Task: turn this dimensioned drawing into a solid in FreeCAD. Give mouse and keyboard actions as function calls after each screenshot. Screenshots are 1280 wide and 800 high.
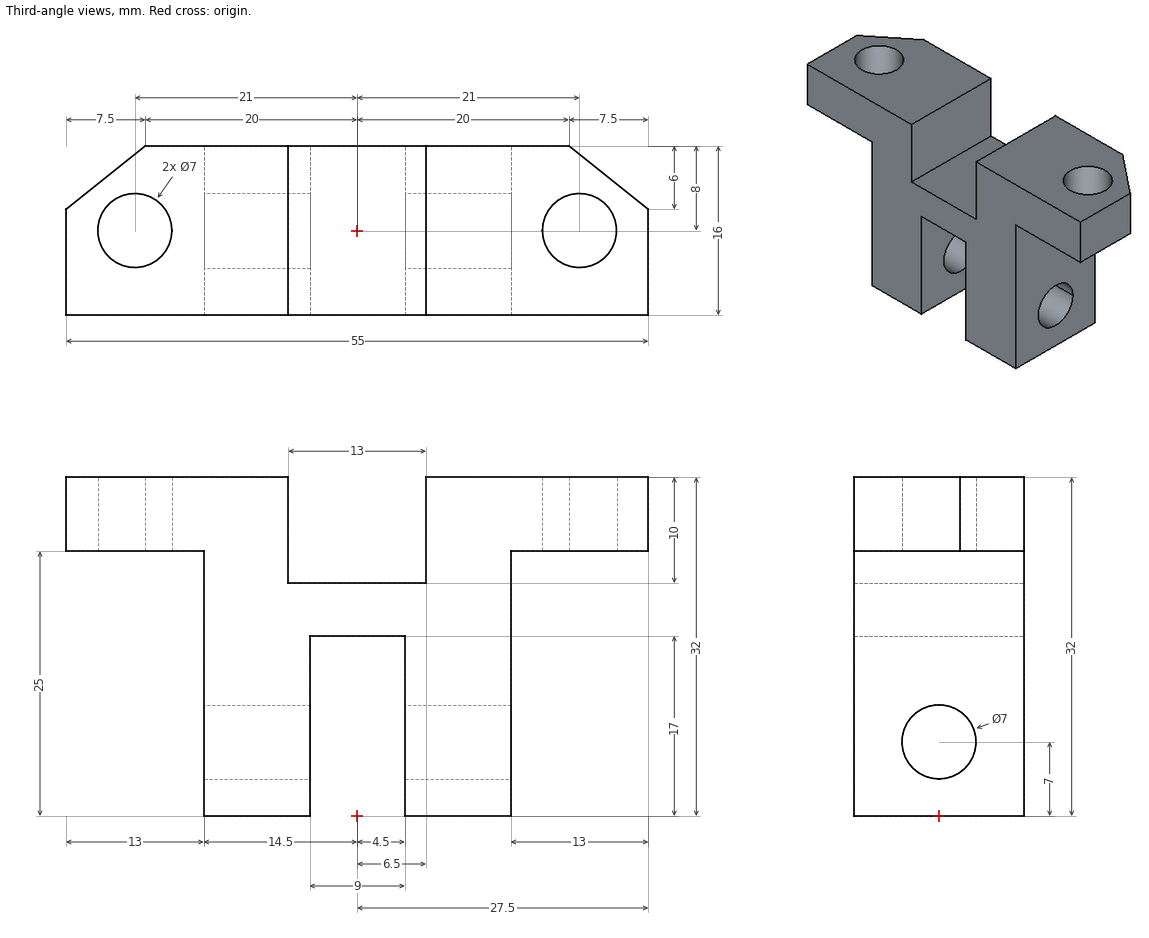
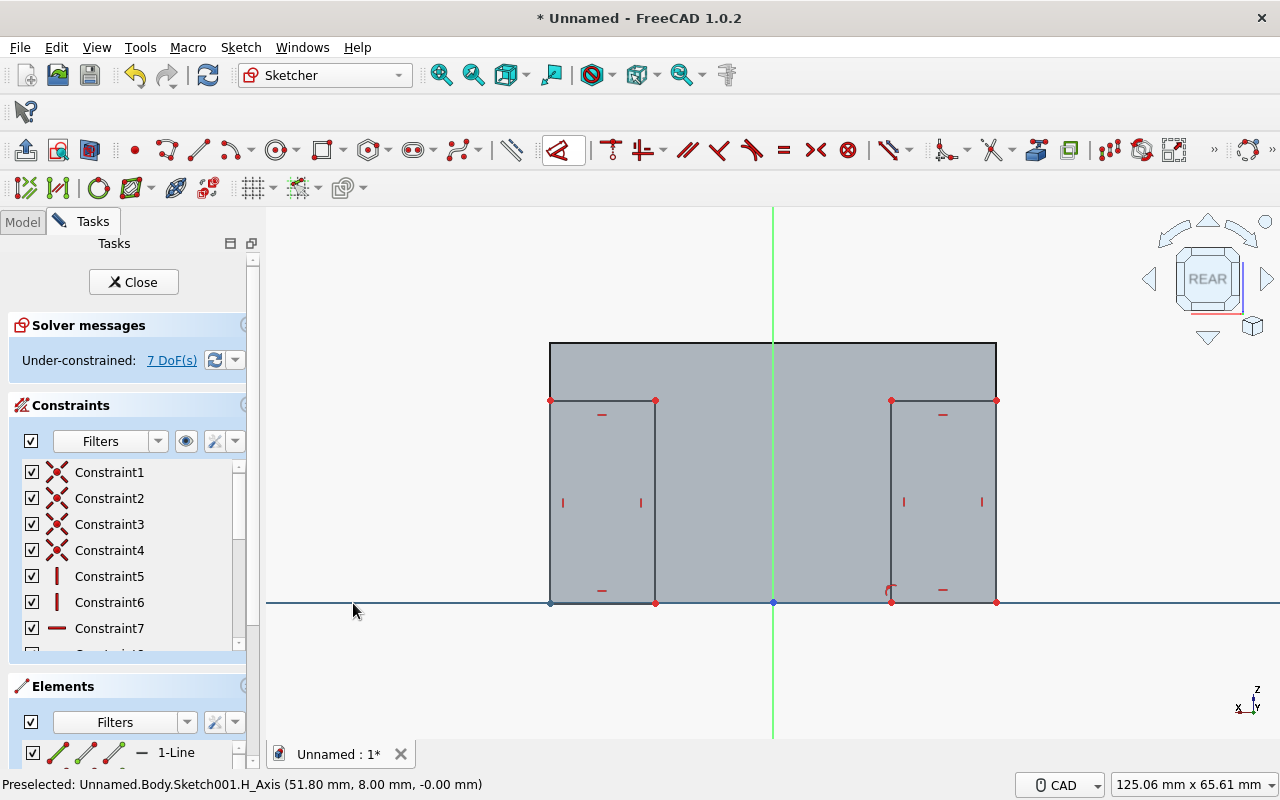
click(612, 150)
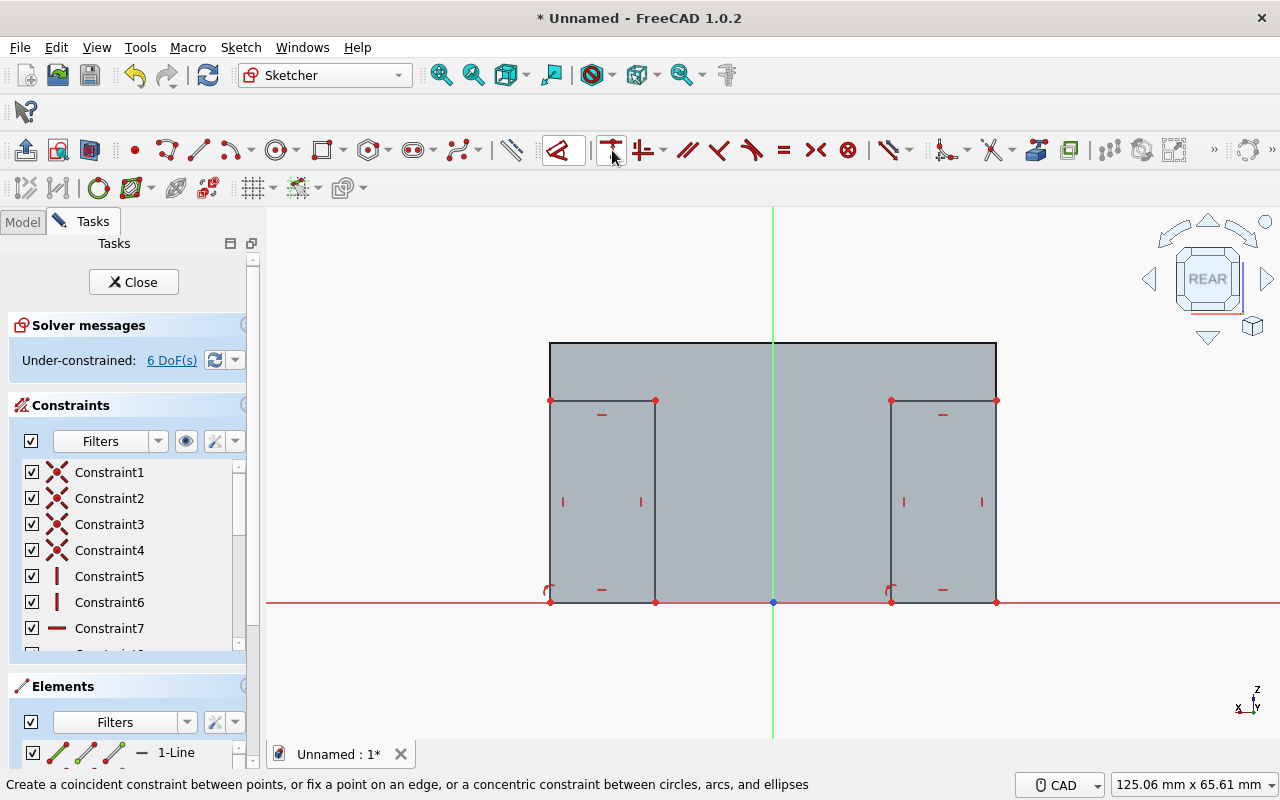
click(891, 462)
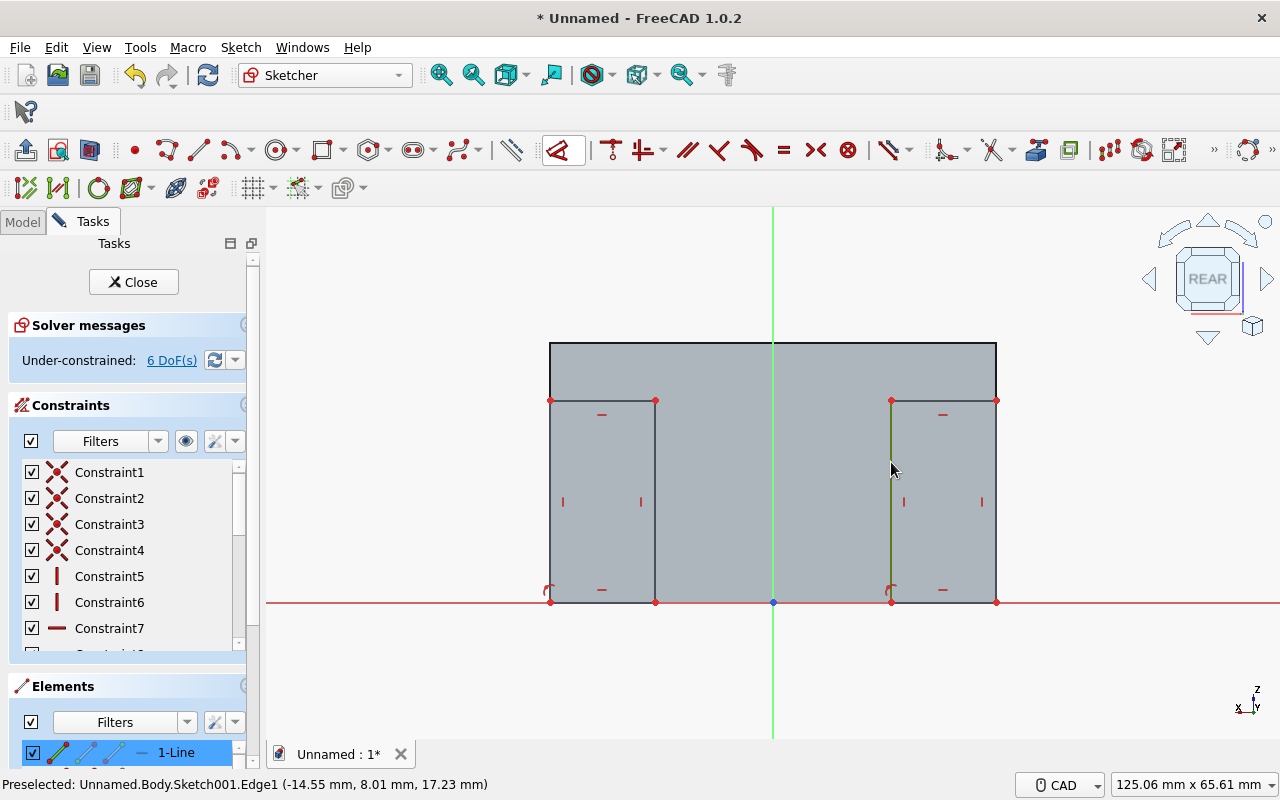
key(i)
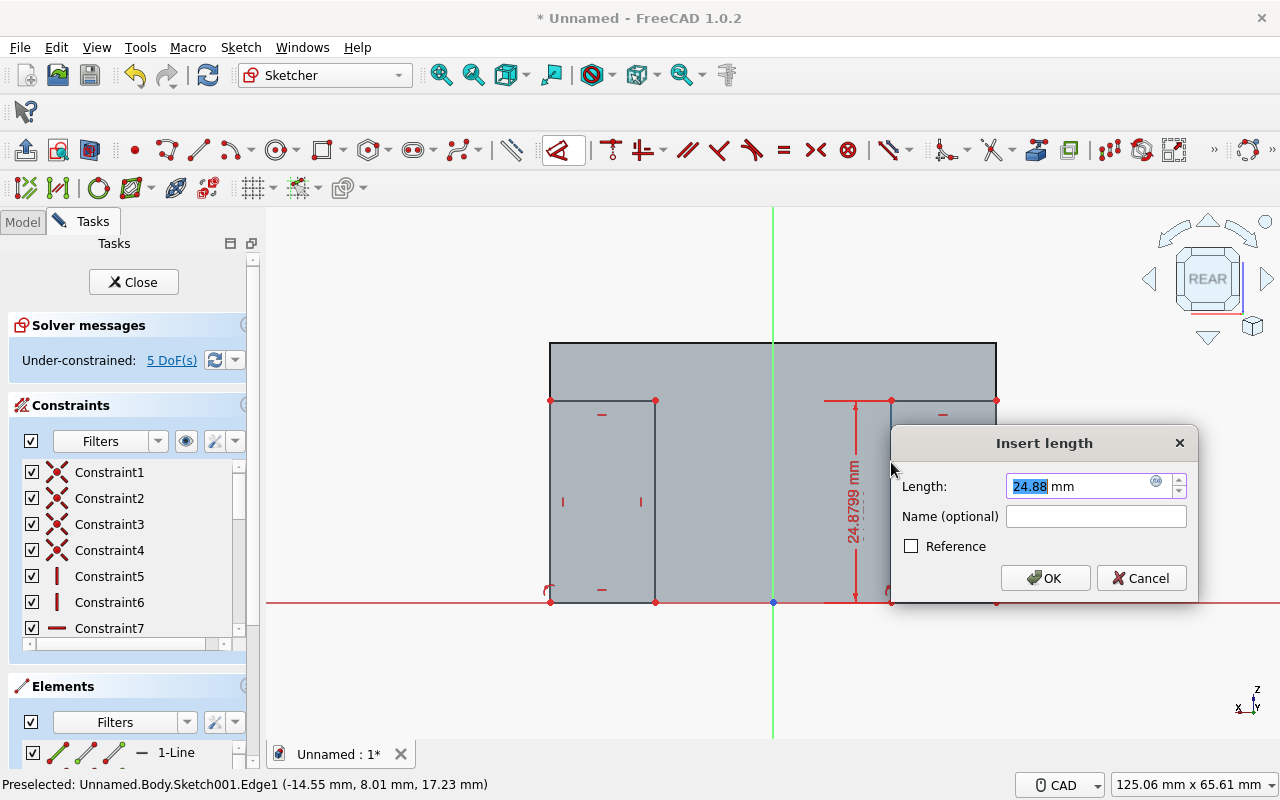
text(25)
key(Return)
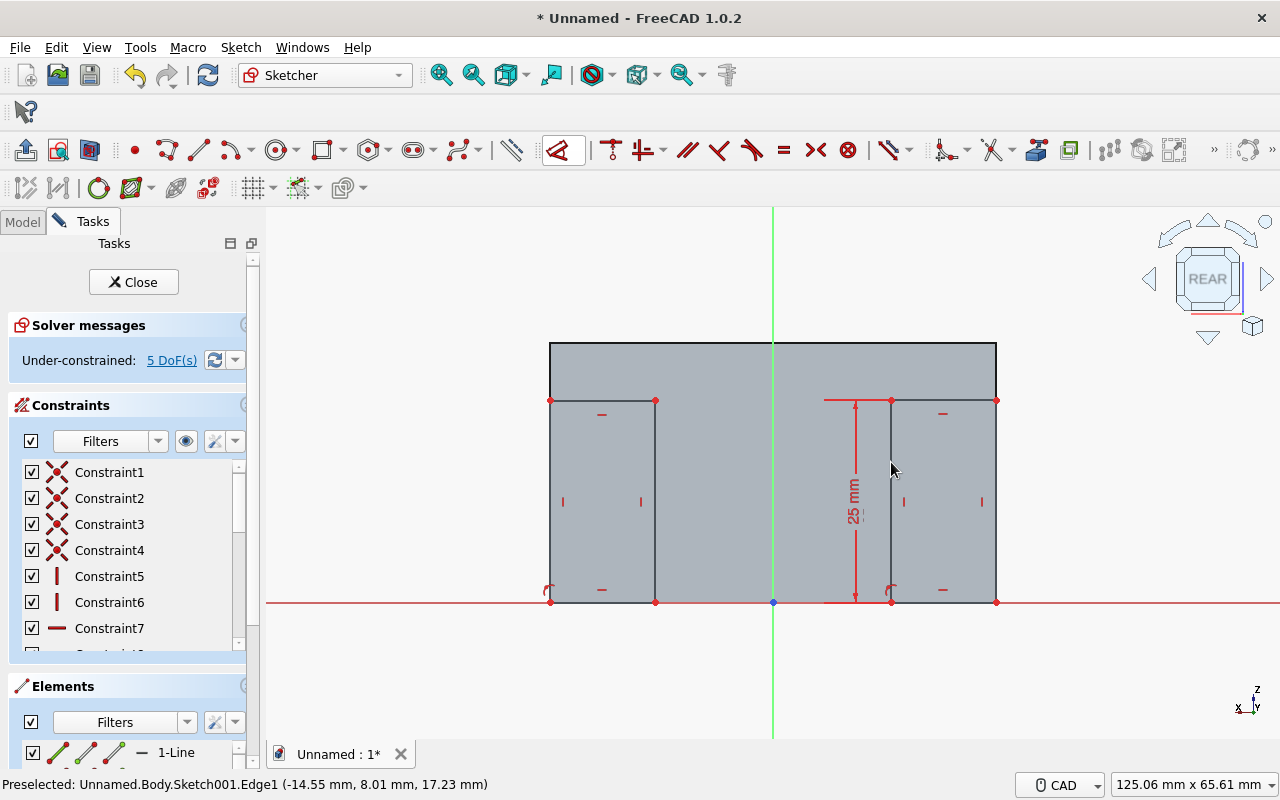
click(922, 603)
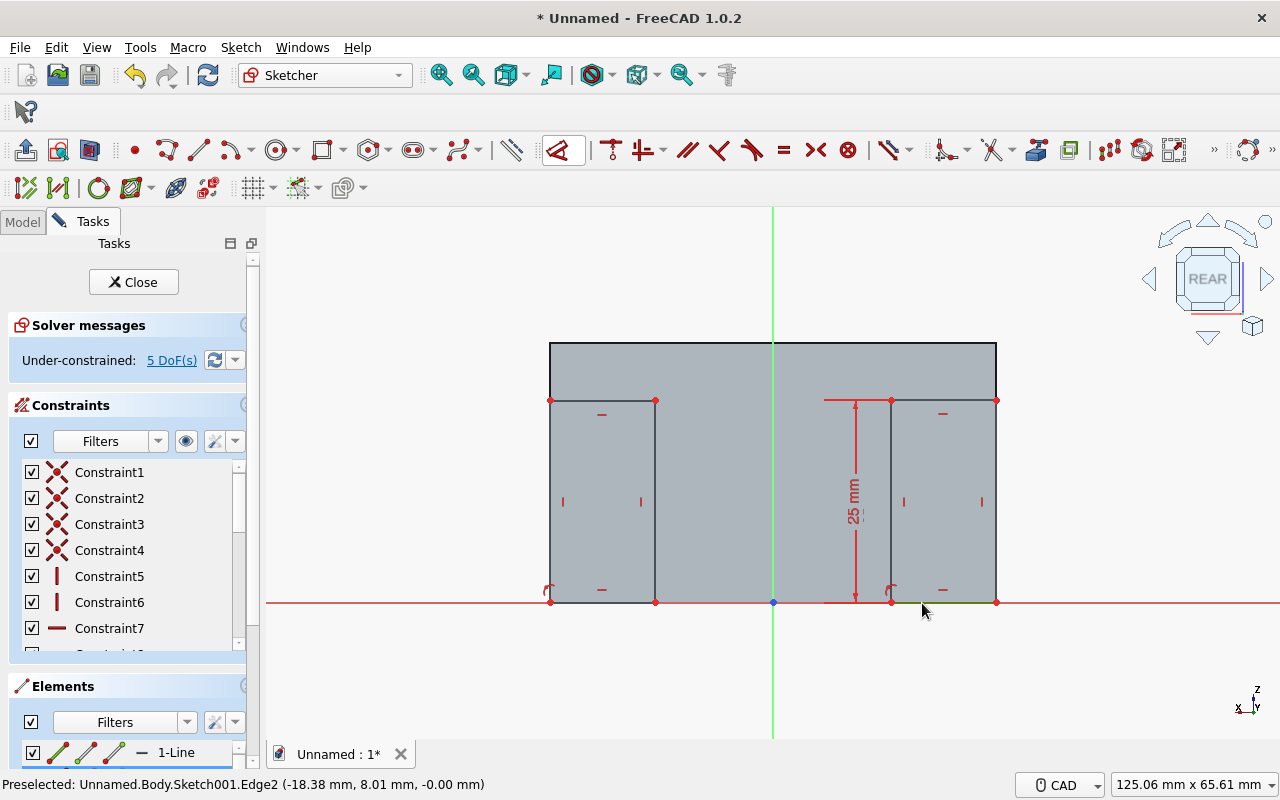
click(580, 150)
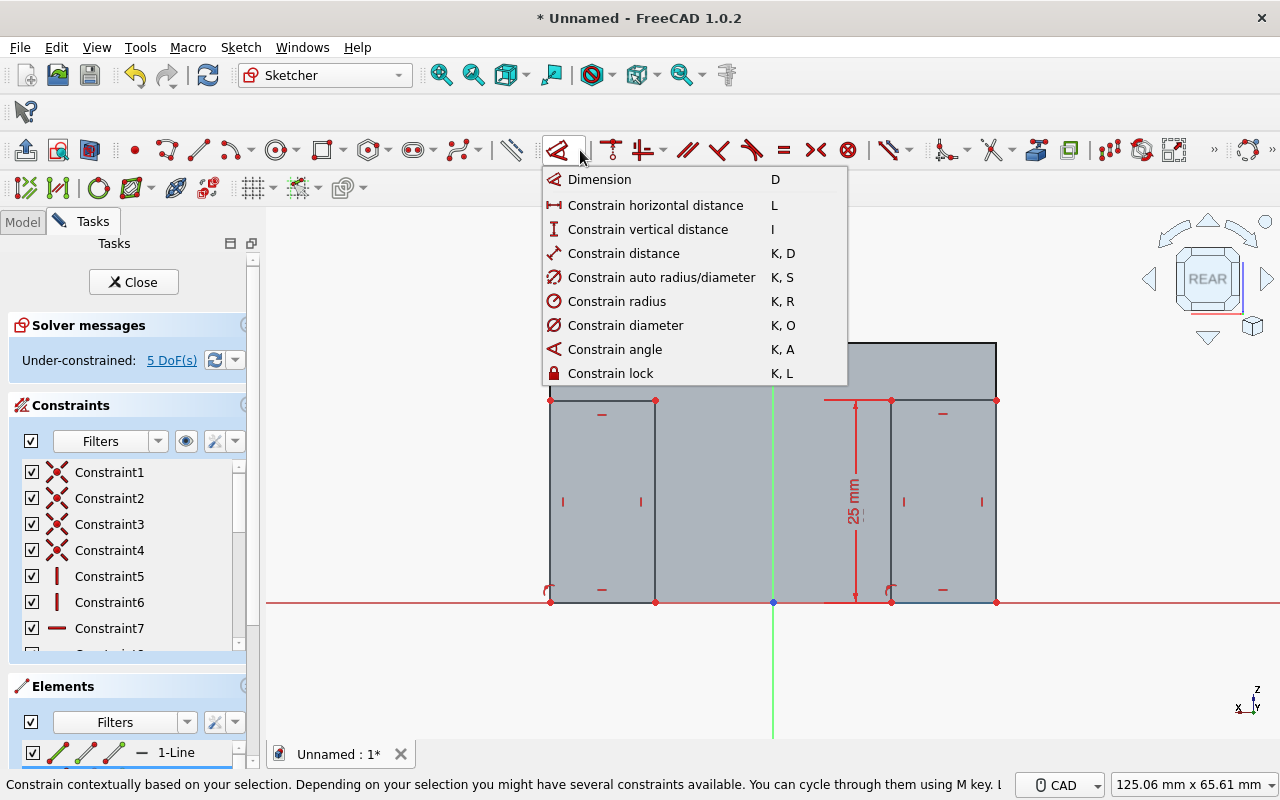
click(695, 205)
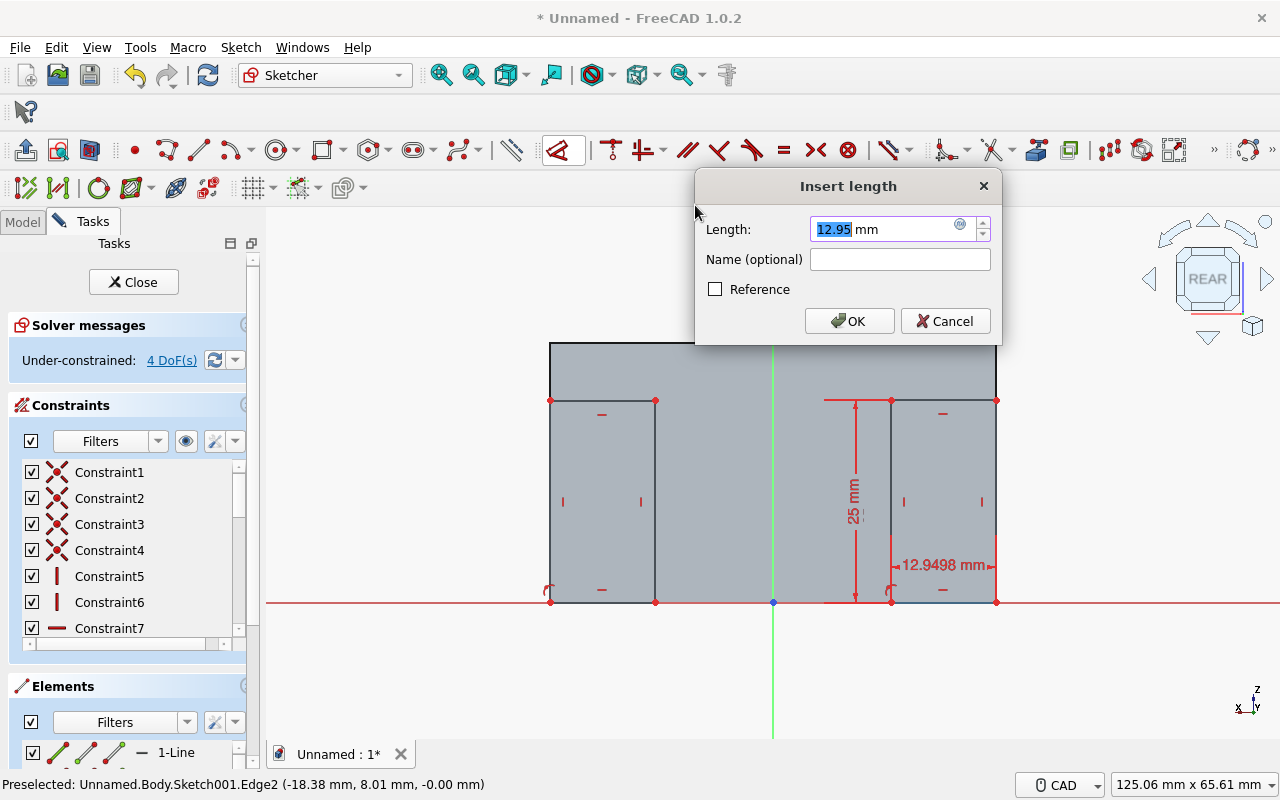
text(13)
key(Return)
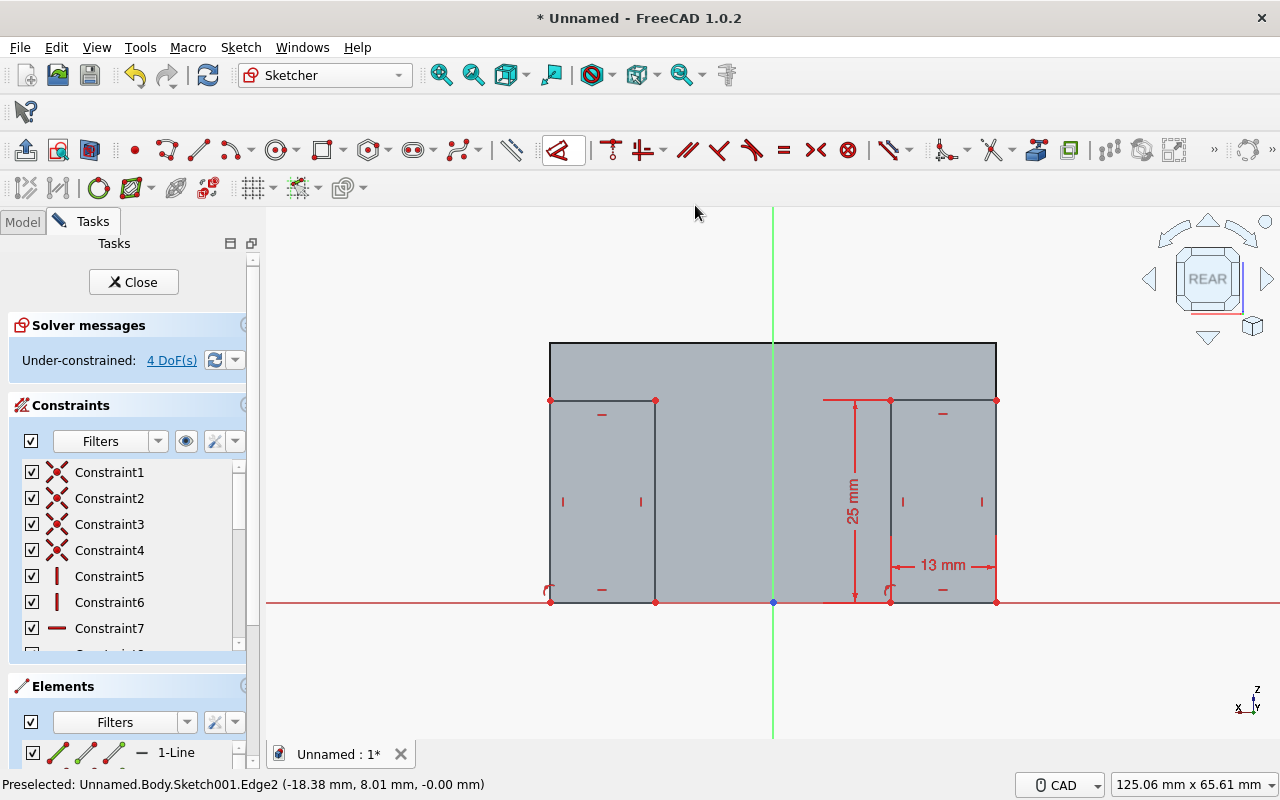
click(550, 462)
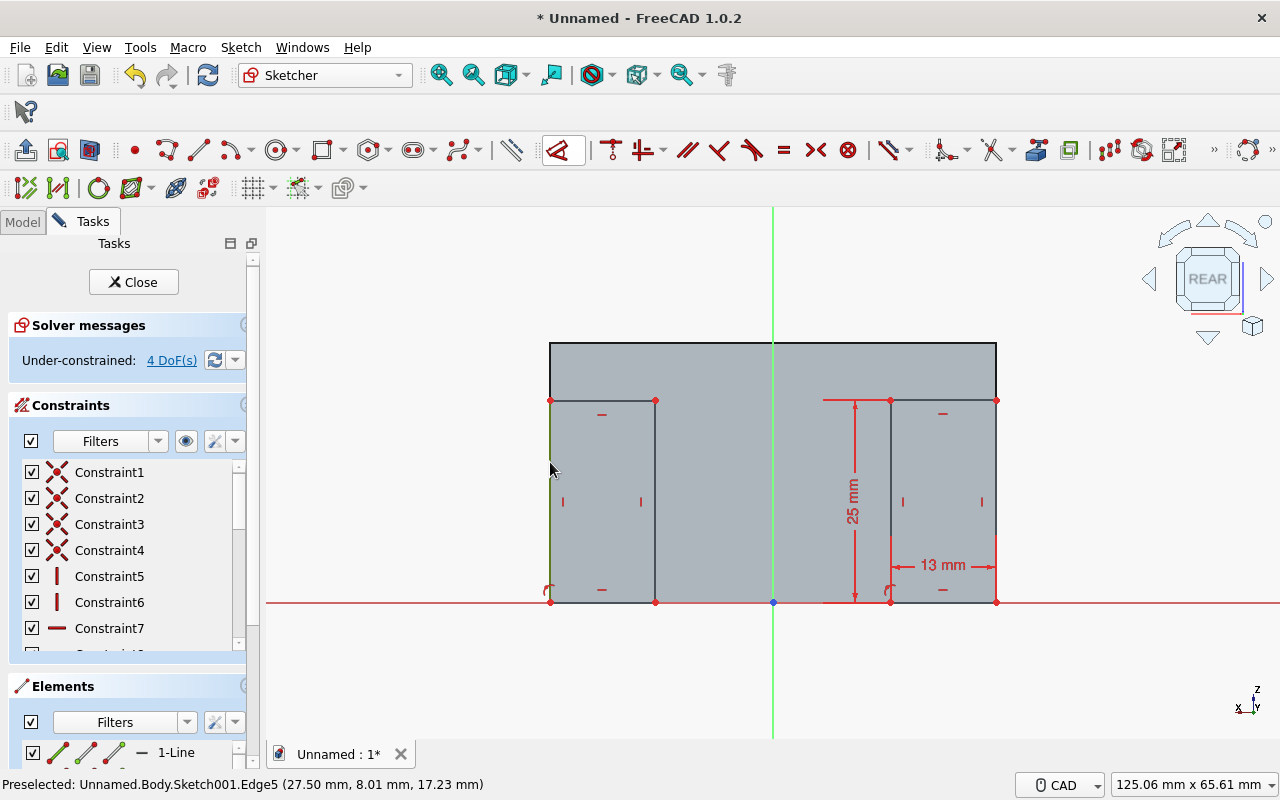
key(i)